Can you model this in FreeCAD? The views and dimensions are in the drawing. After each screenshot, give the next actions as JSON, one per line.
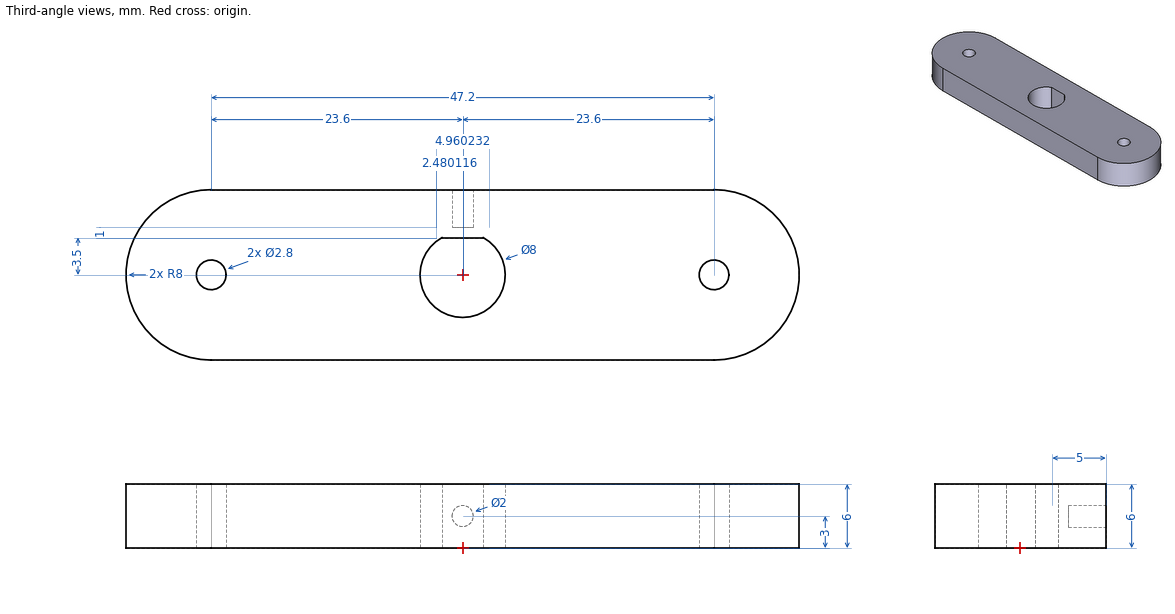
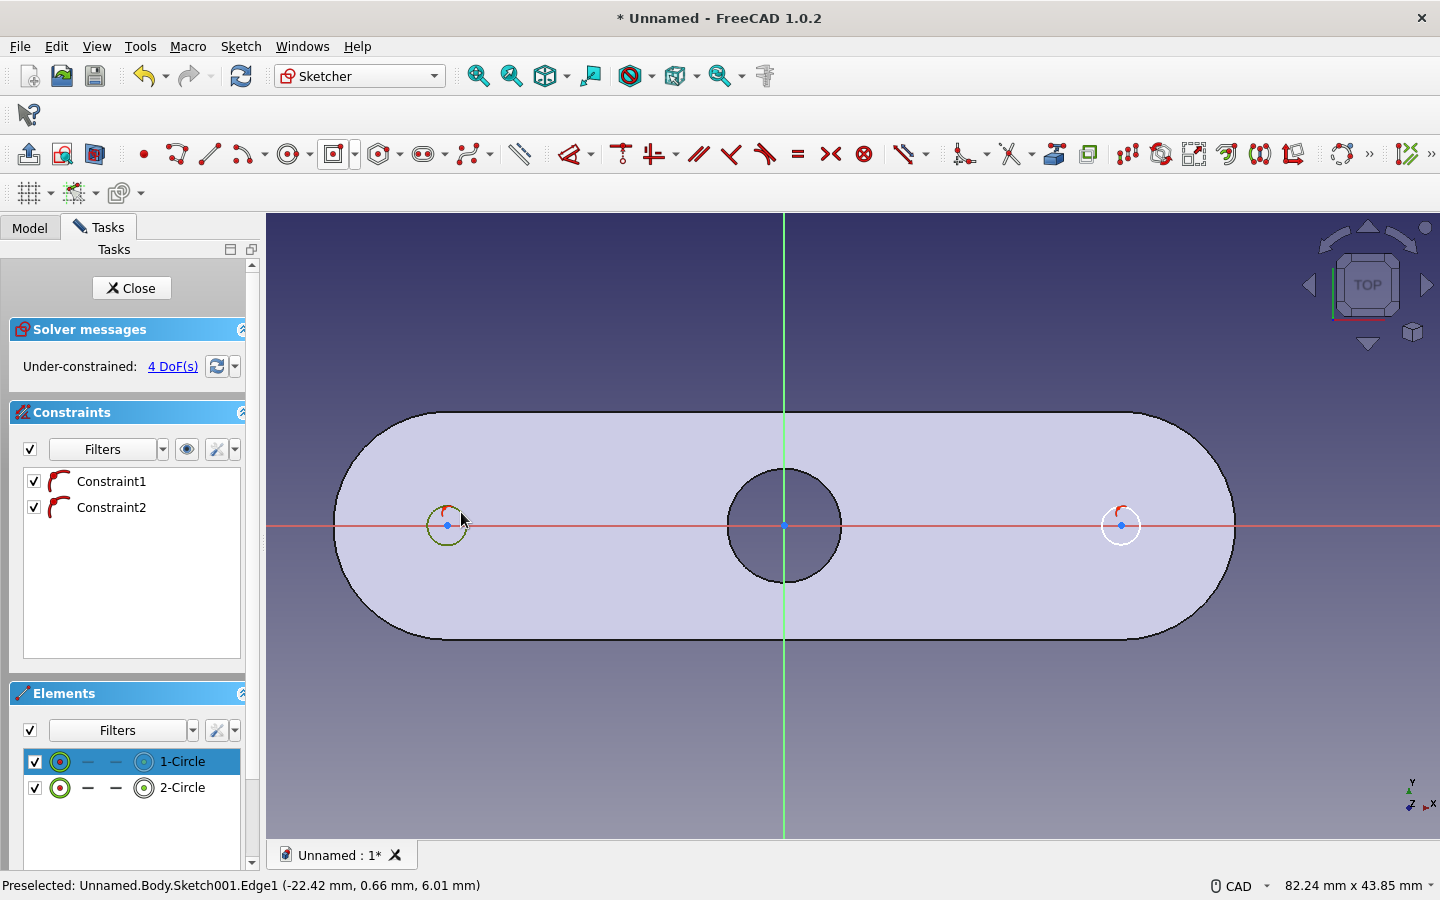
{"action": "left_click", "coordinate": [1134, 512]}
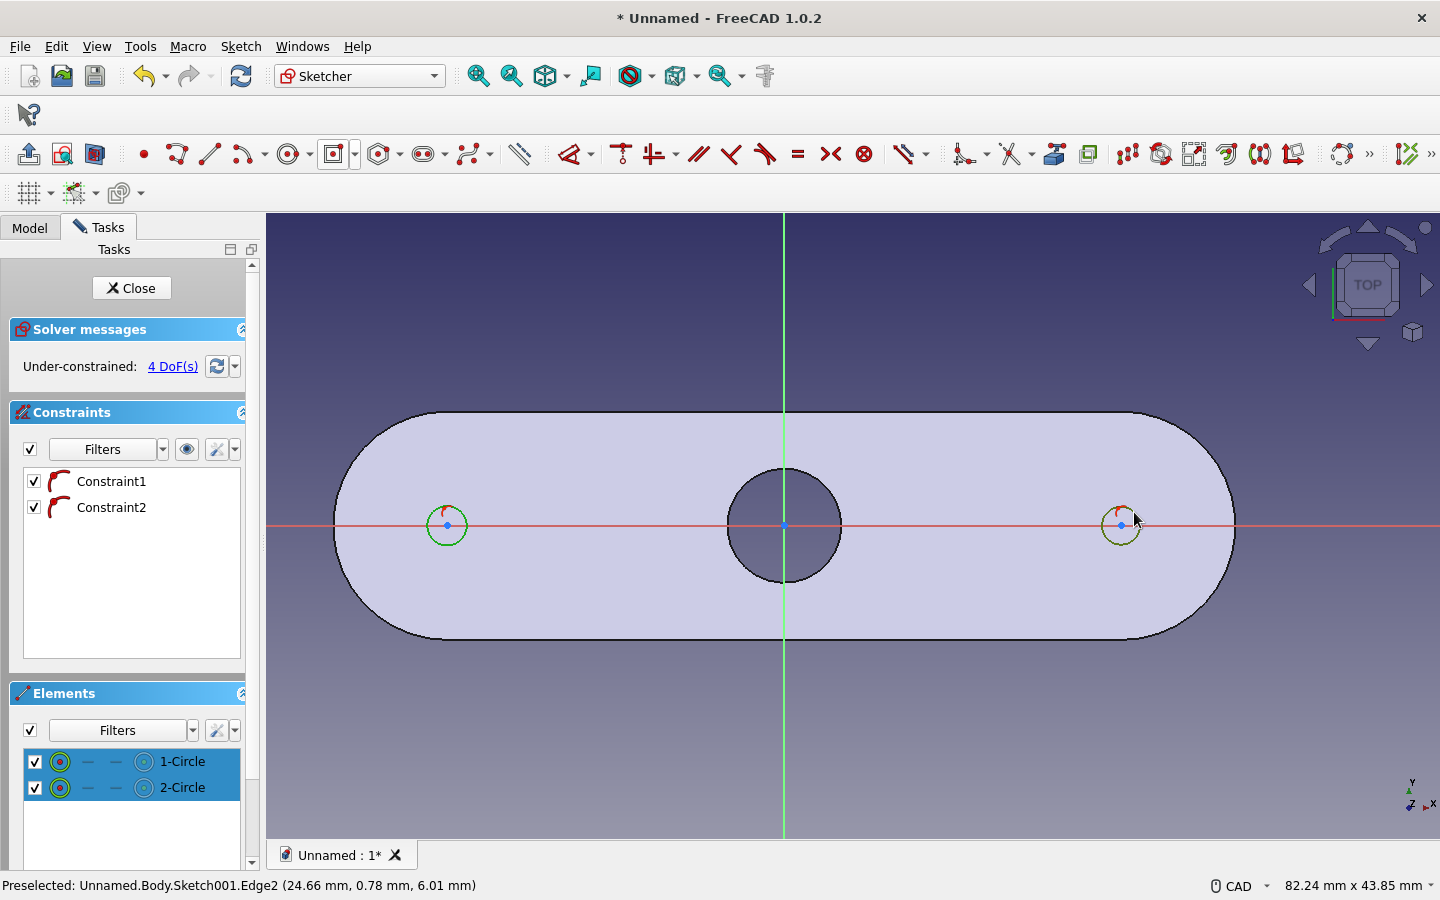
{"action": "left_click", "coordinate": [798, 154]}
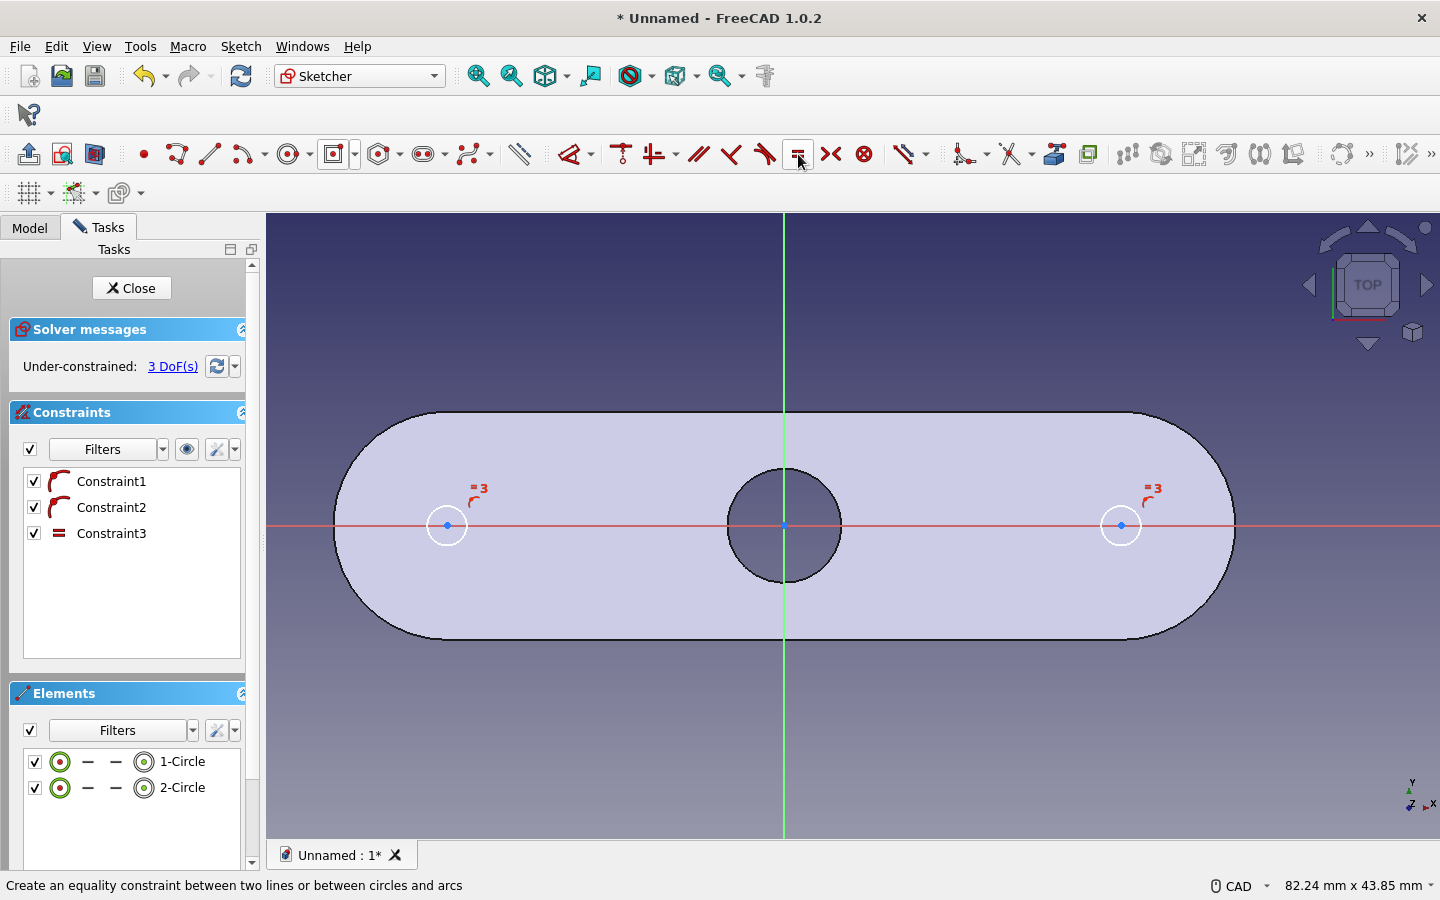
{"action": "left_click", "coordinate": [568, 154]}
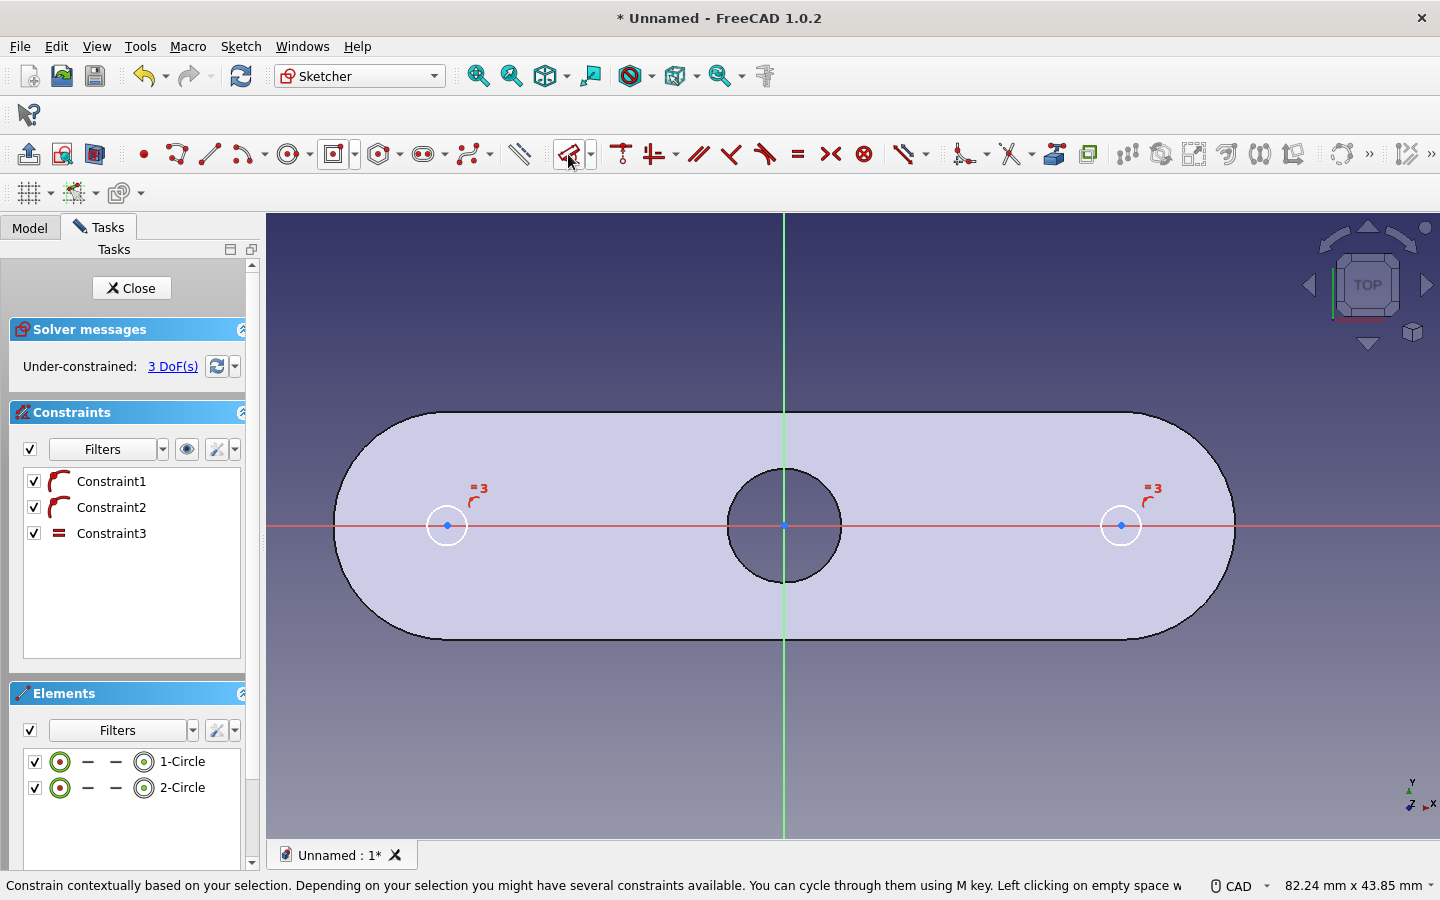
{"action": "left_click", "coordinate": [461, 512]}
{"action": "left_click", "coordinate": [484, 490]}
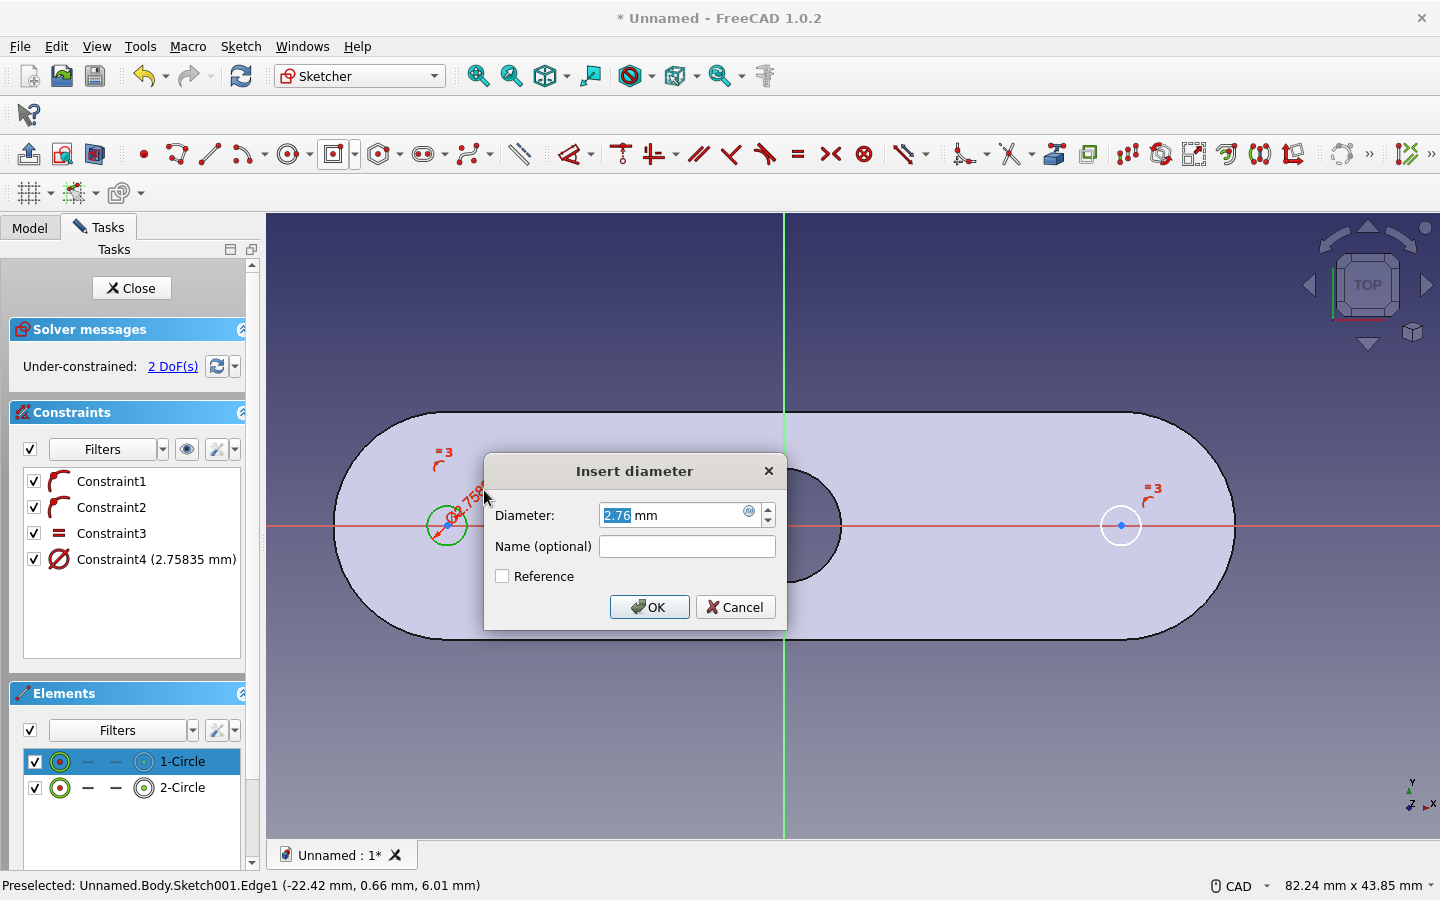
{"action": "type", "text": "2.8"}
{"action": "key", "text": "Return"}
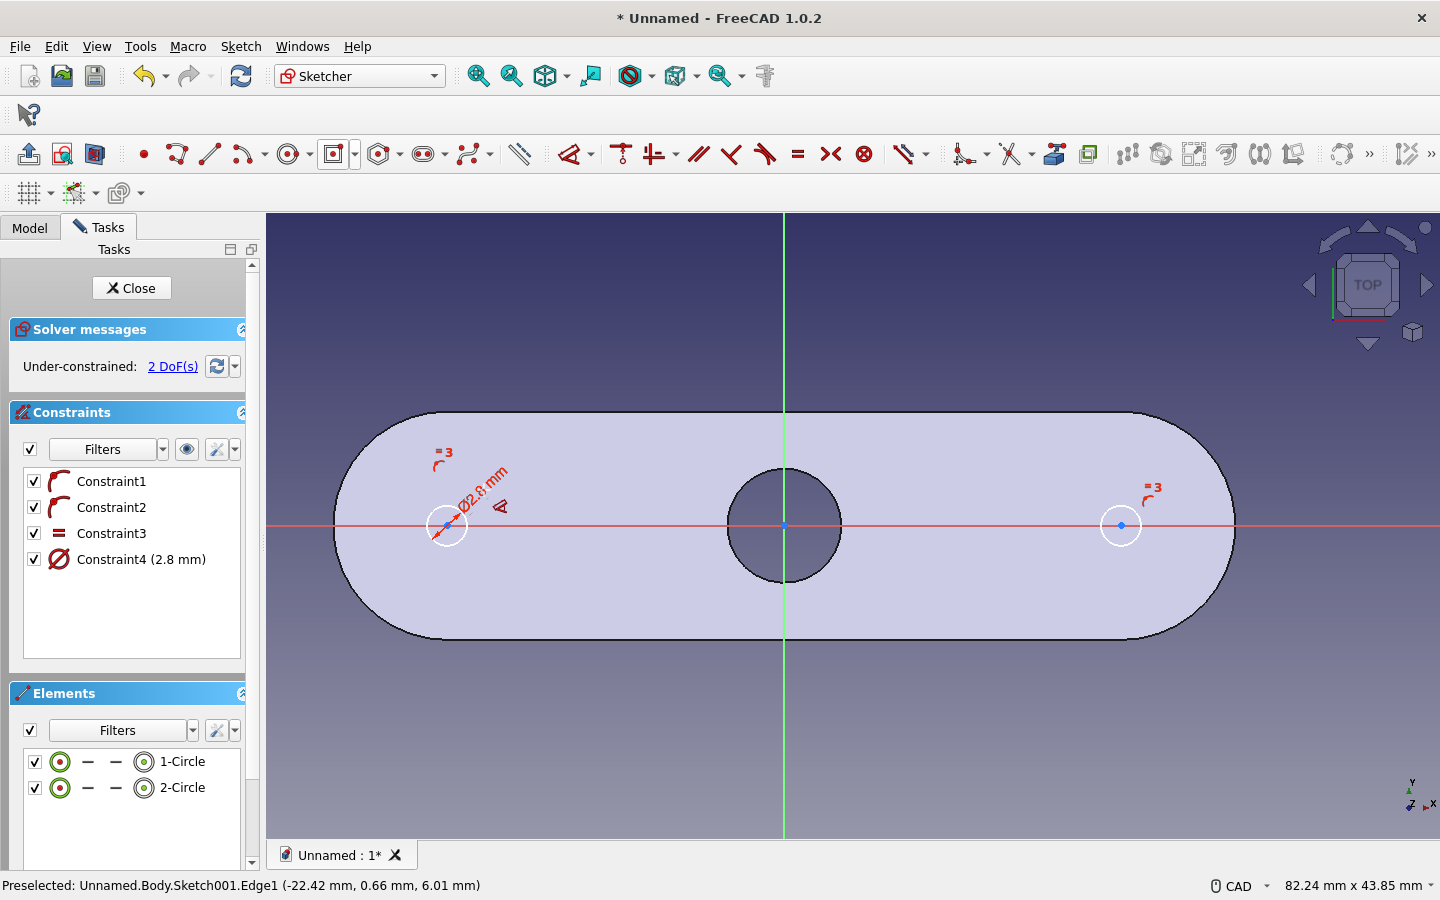
{"action": "left_click", "coordinate": [447, 526]}
{"action": "left_click", "coordinate": [616, 560]}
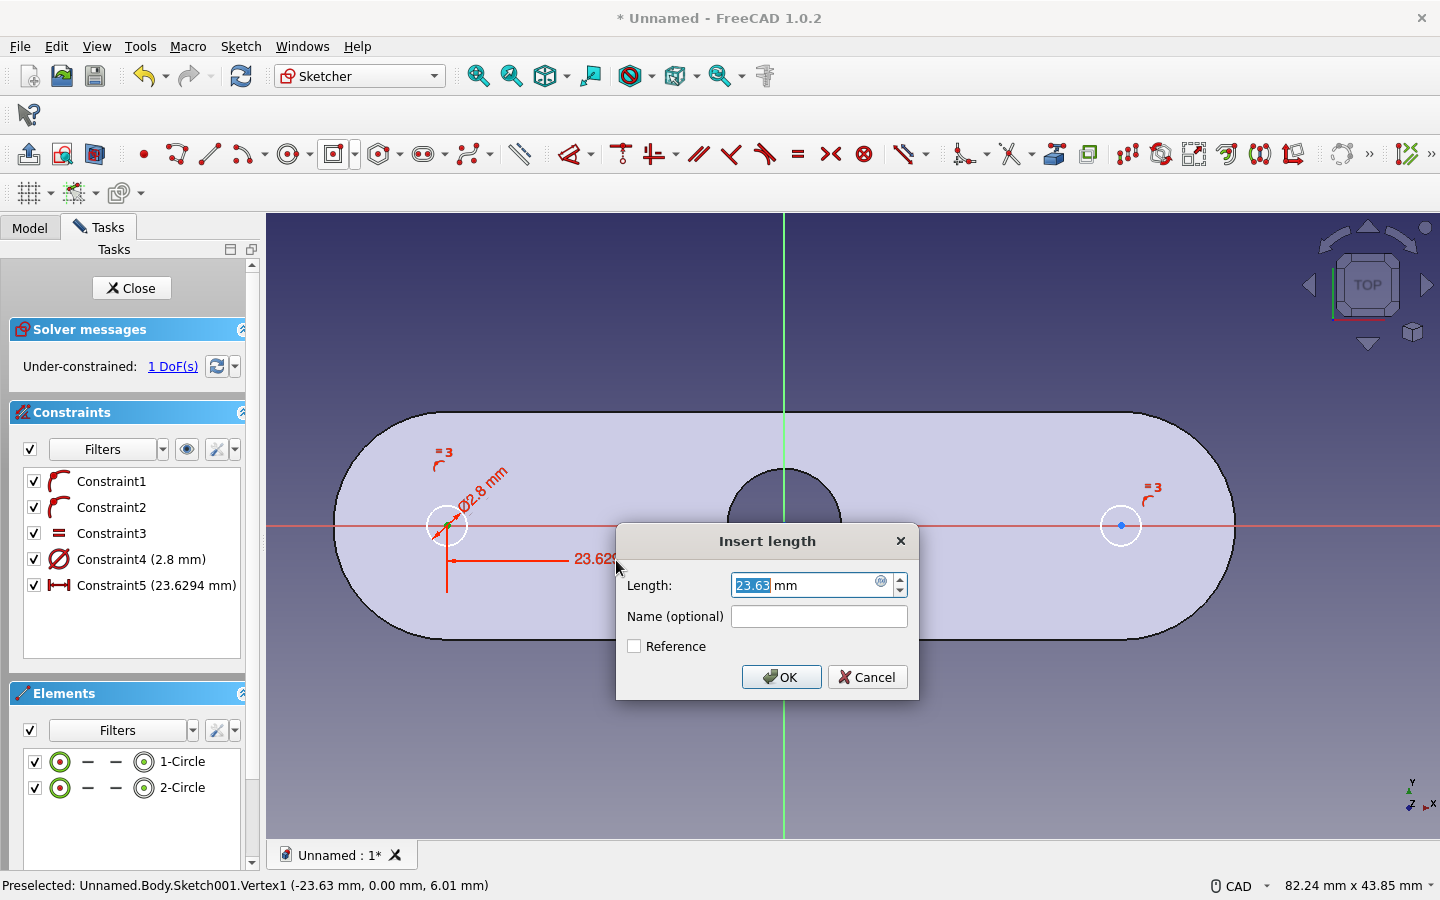
{"action": "type", "text": "23.6"}
{"action": "key", "text": "Return"}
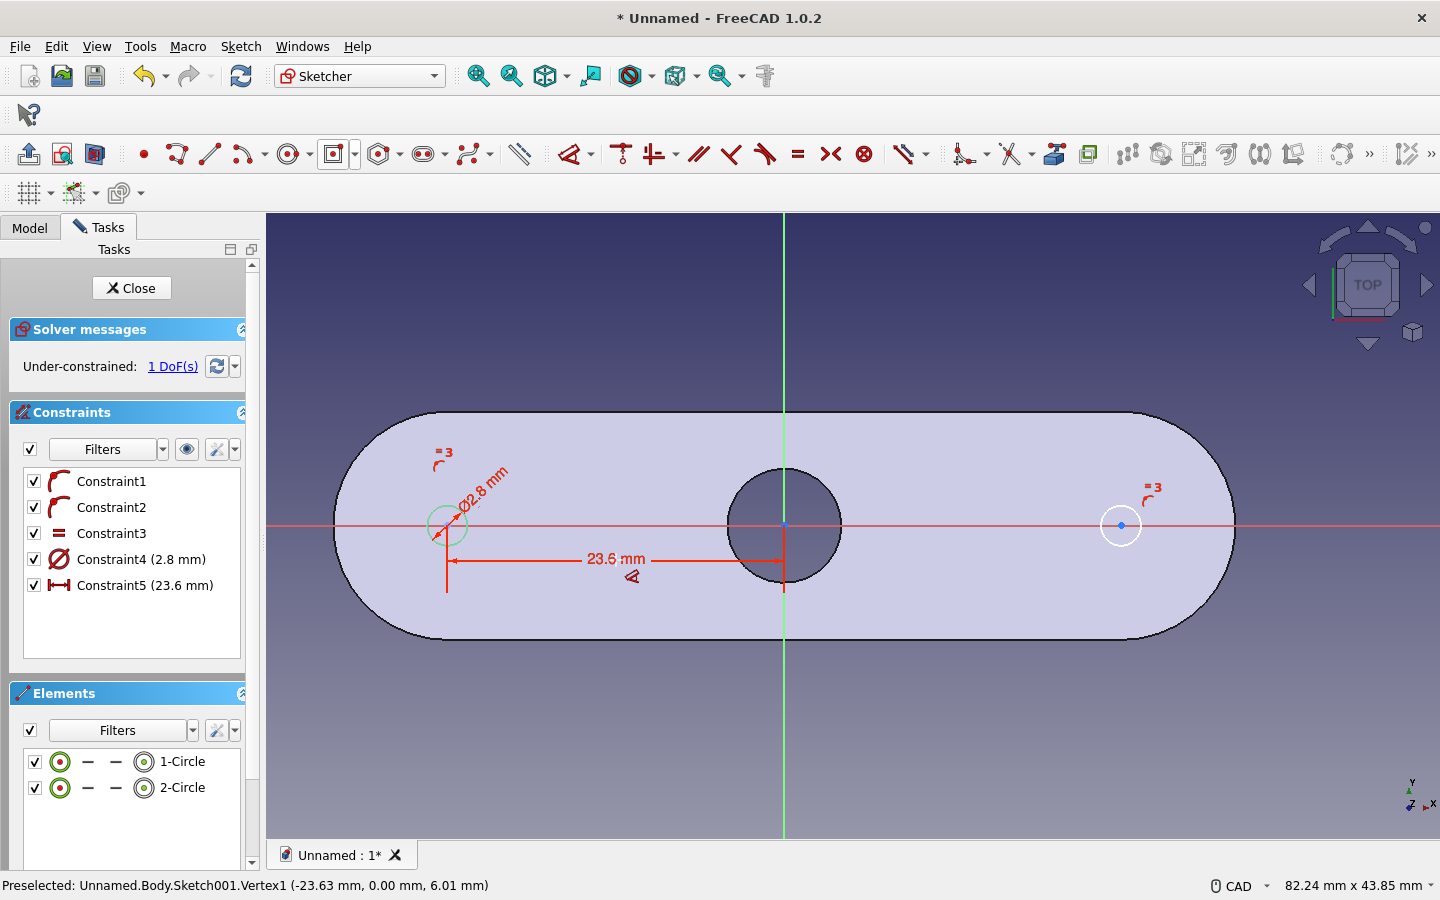
{"action": "left_click", "coordinate": [1121, 526]}
{"action": "left_click", "coordinate": [953, 560]}